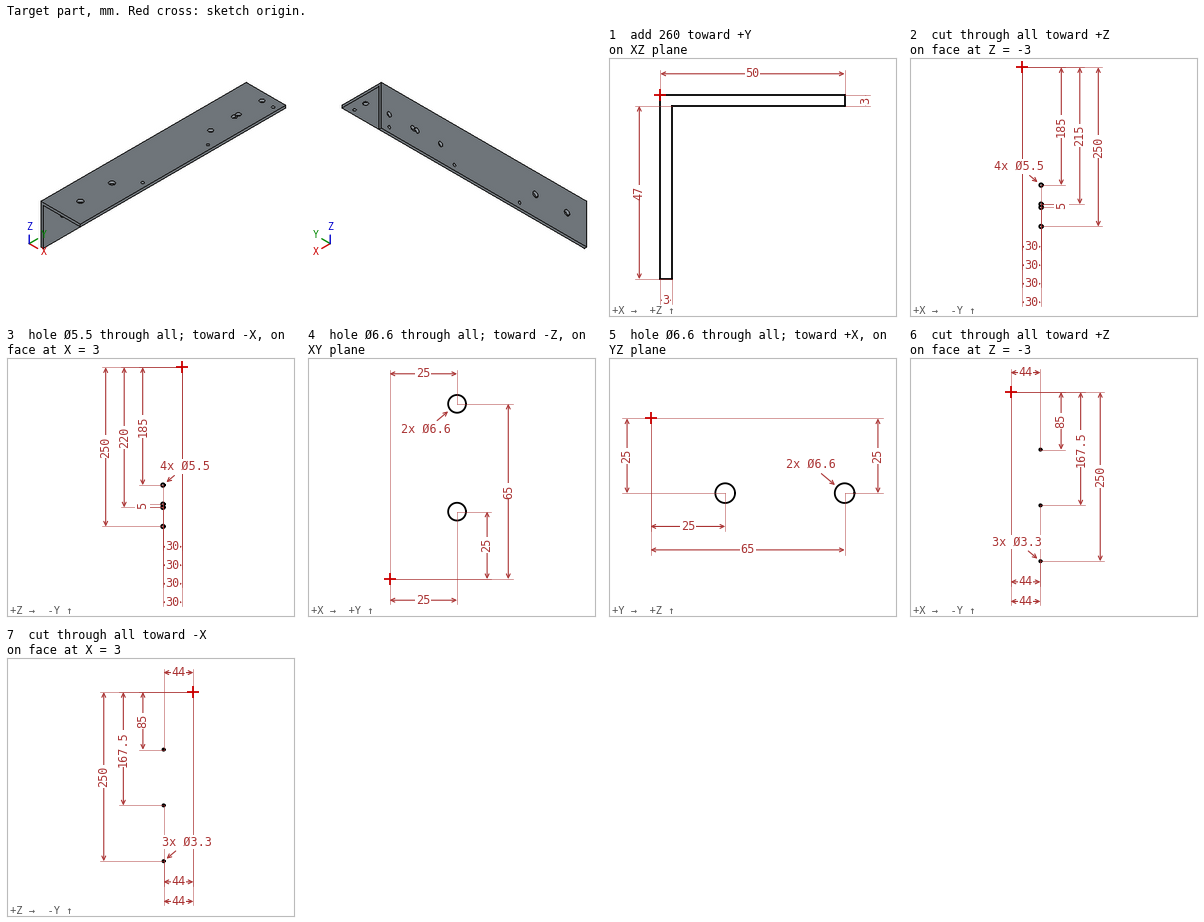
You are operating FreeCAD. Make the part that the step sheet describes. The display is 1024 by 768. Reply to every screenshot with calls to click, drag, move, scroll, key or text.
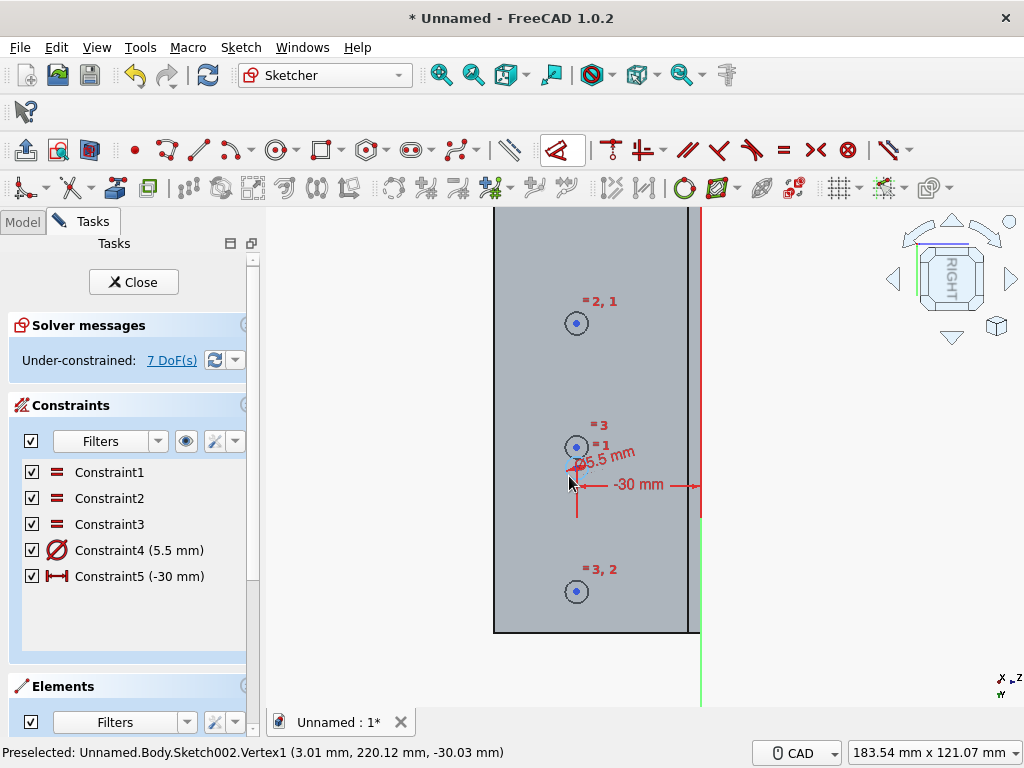
click(577, 324)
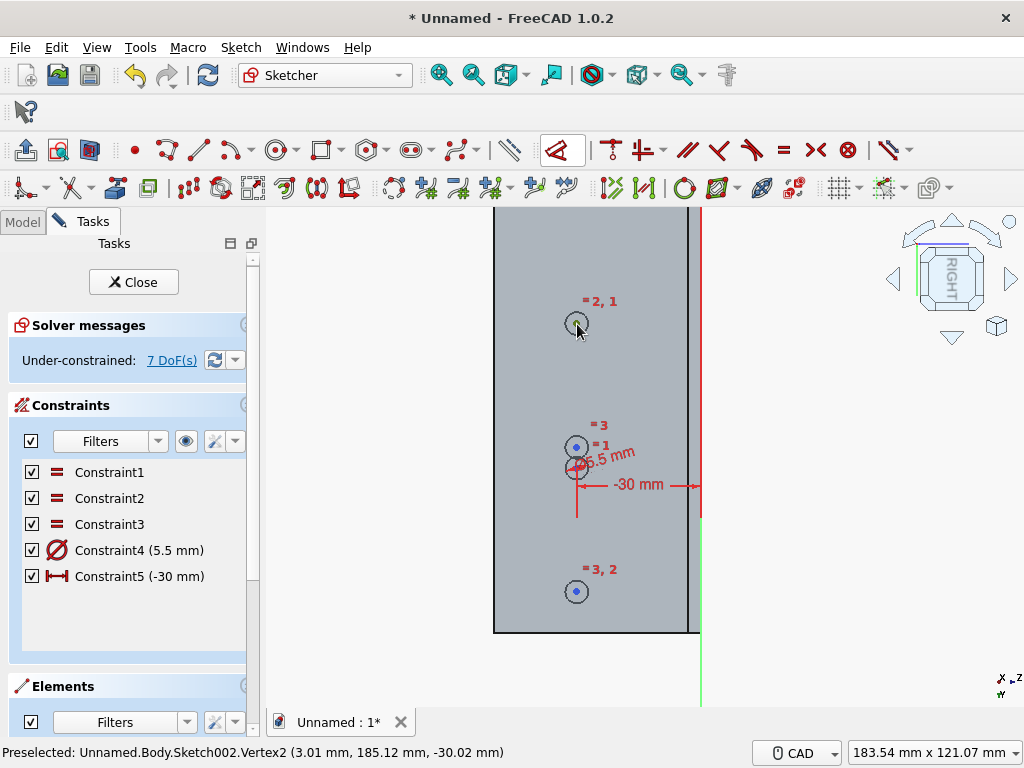
key(l)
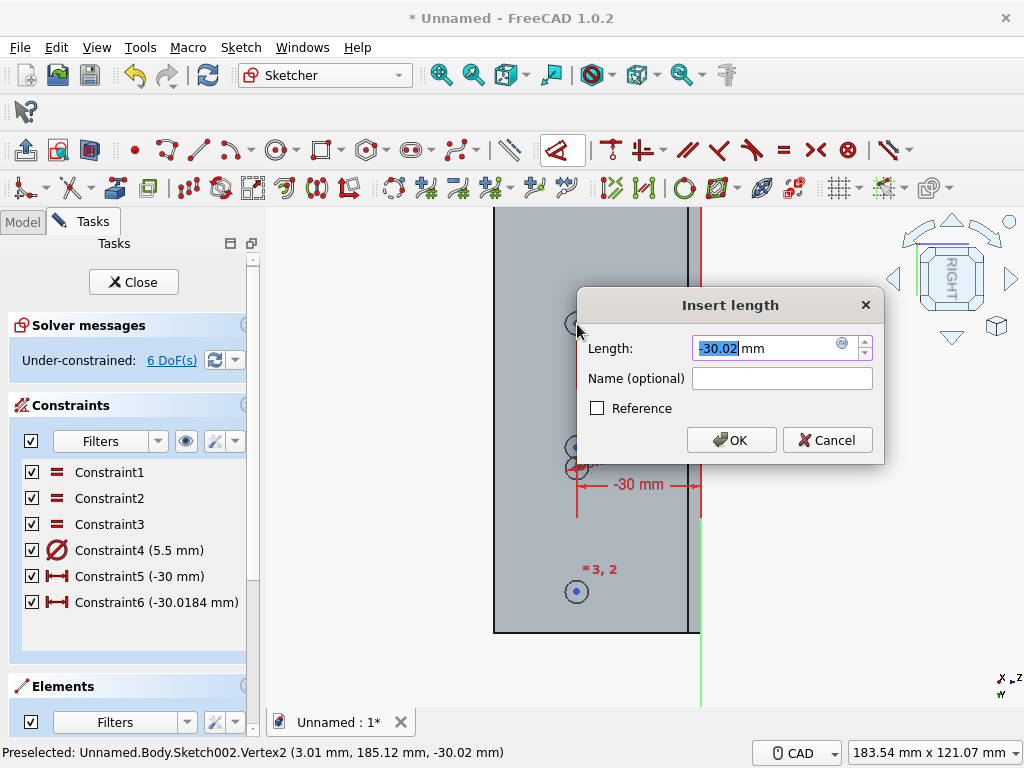
text(-30)
key(Return)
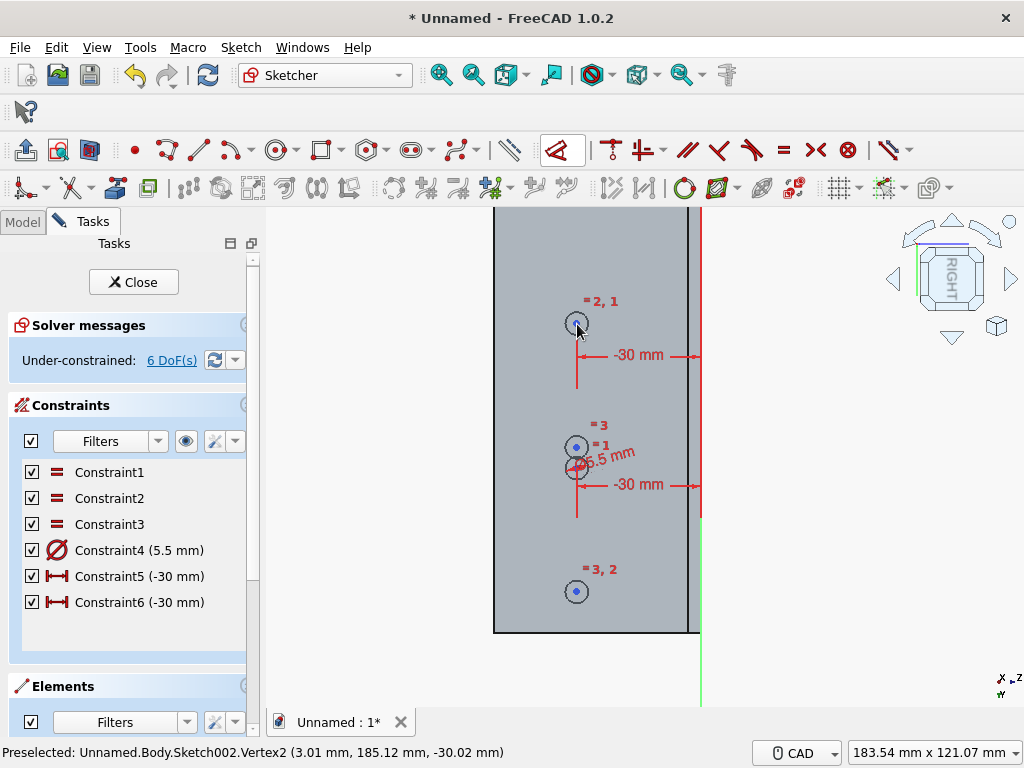
click(577, 592)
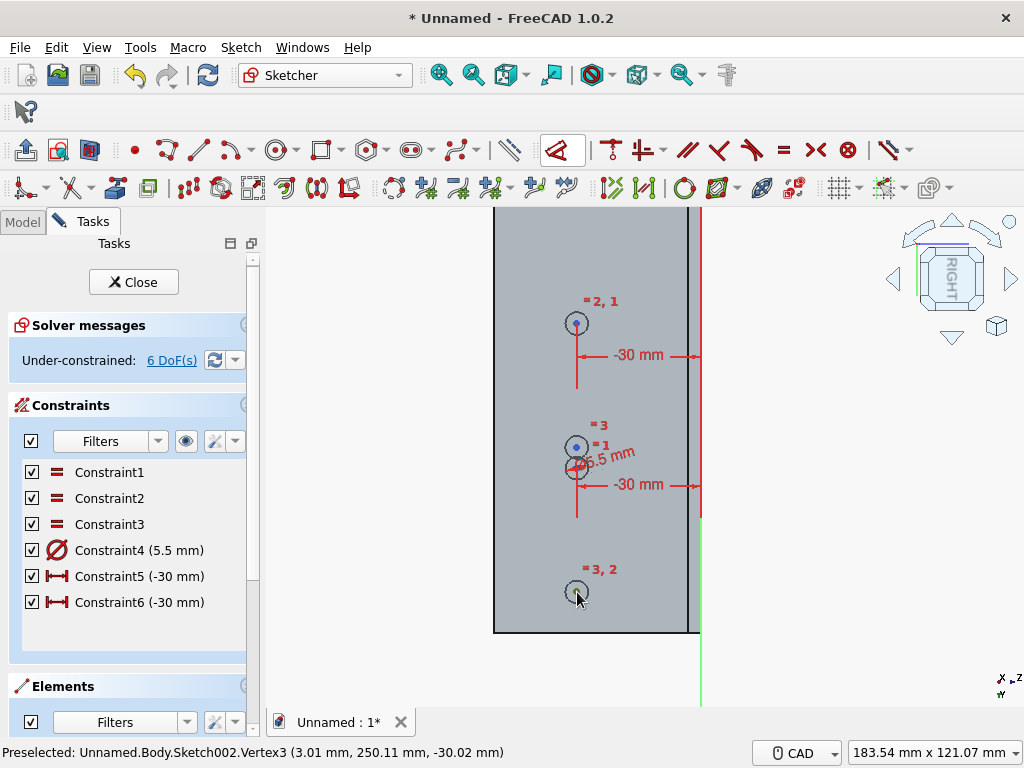
key(l)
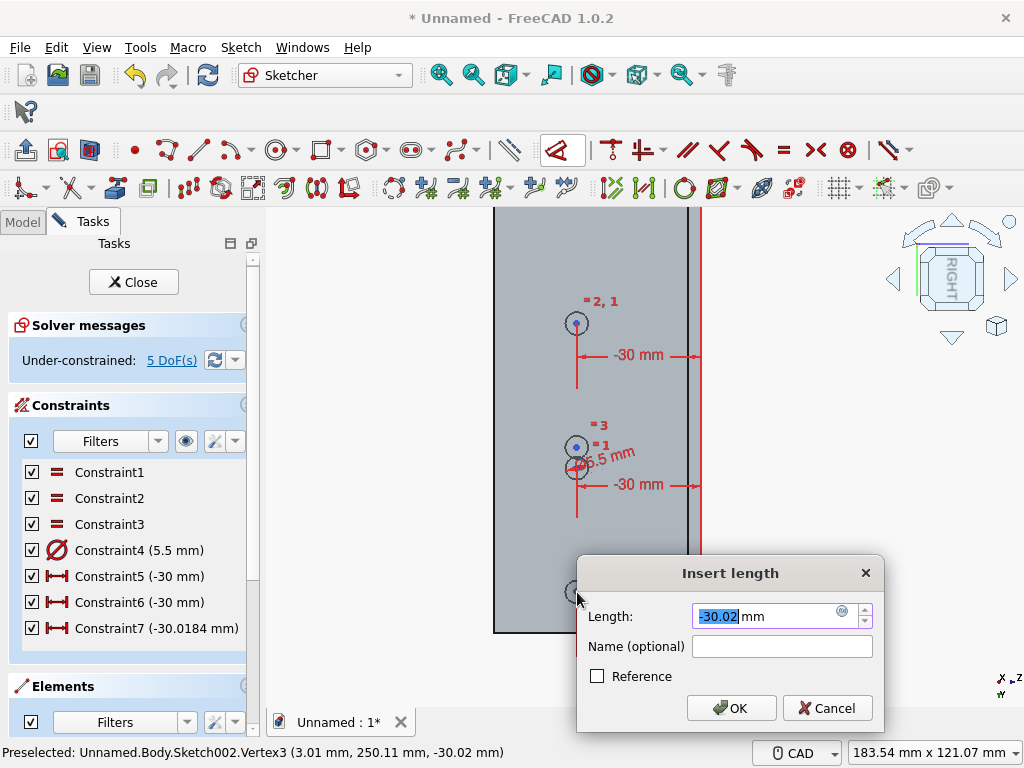
text(-30)
key(Return)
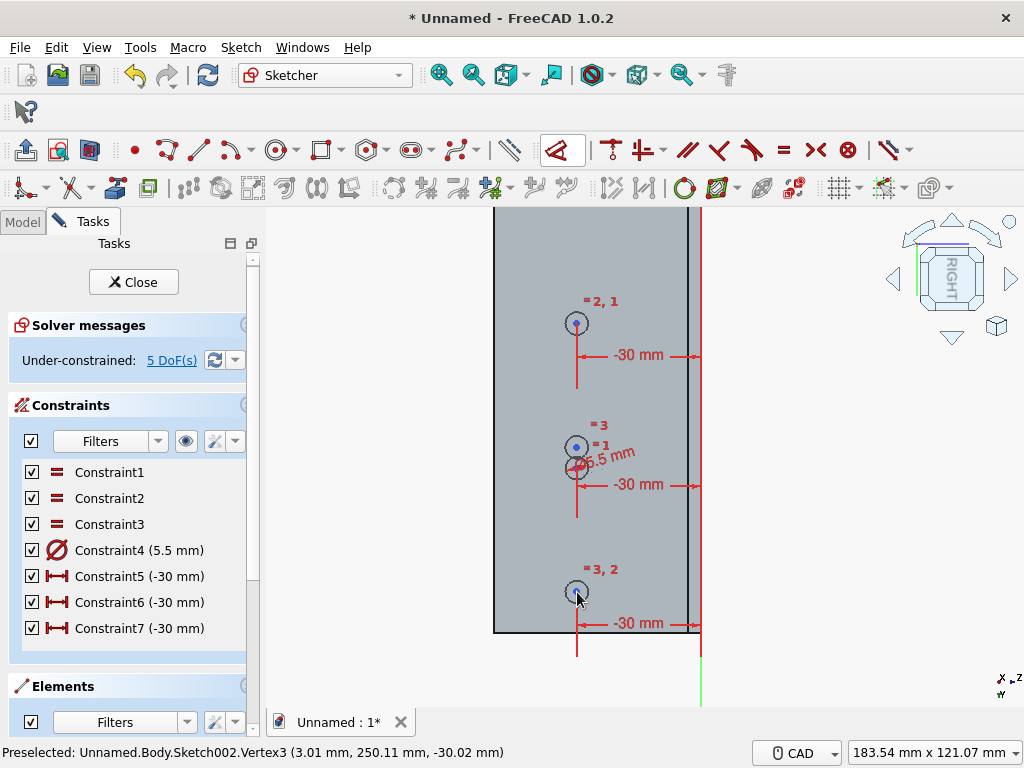
click(577, 447)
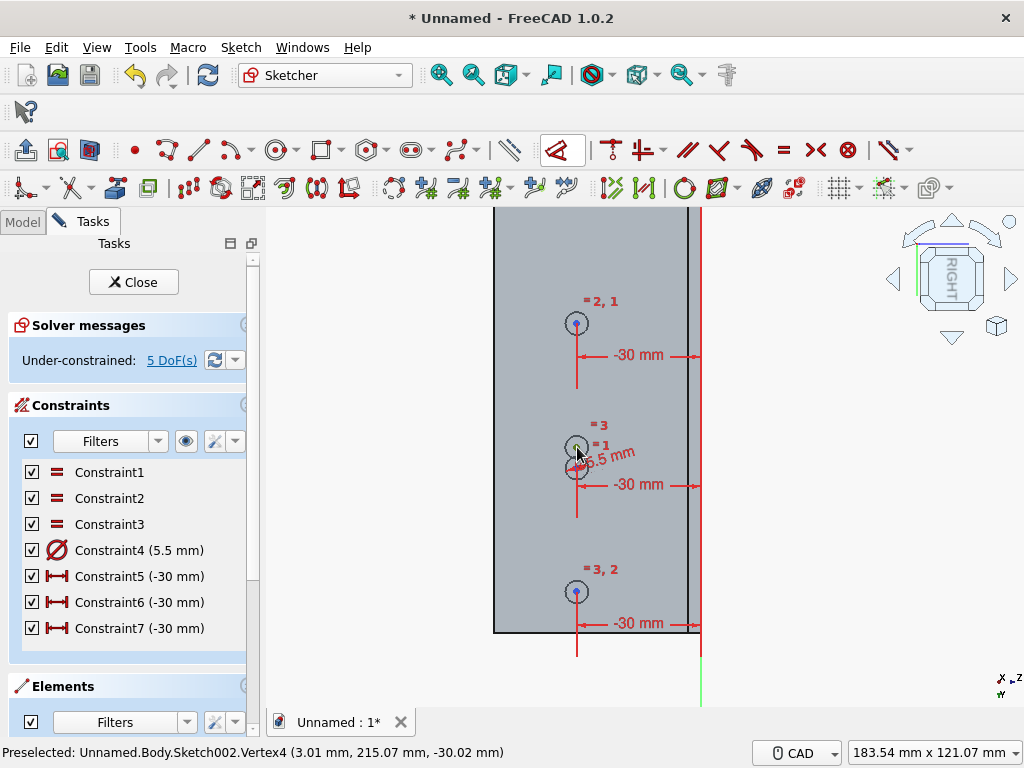
key(l)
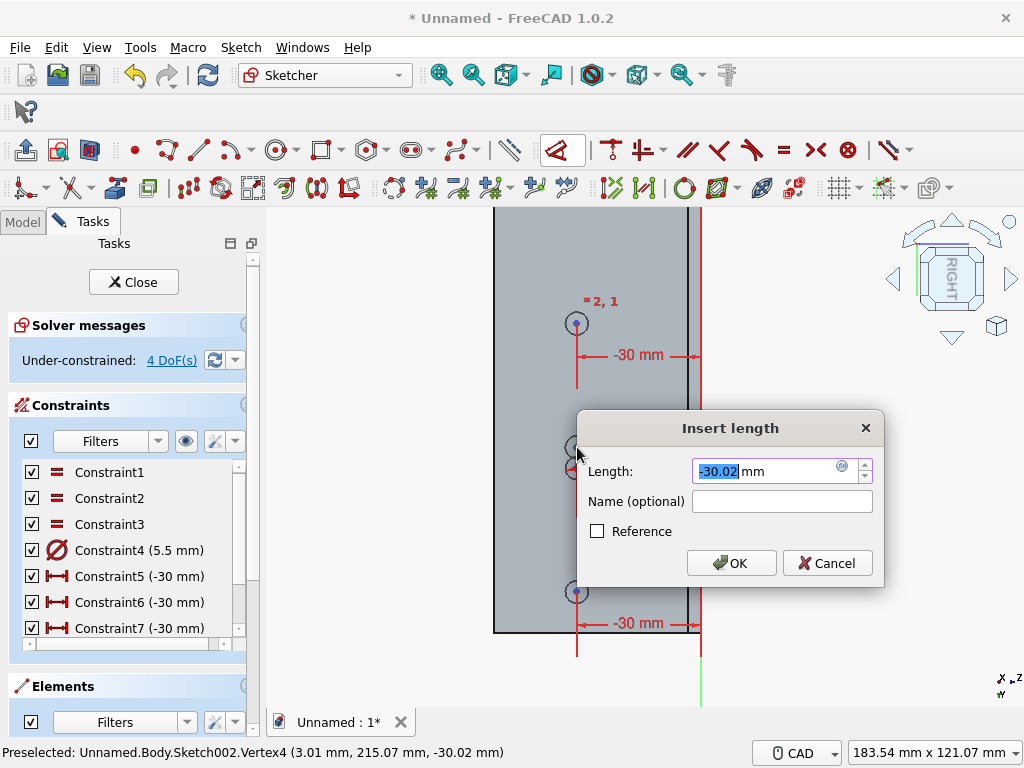
text(-30)
key(Return)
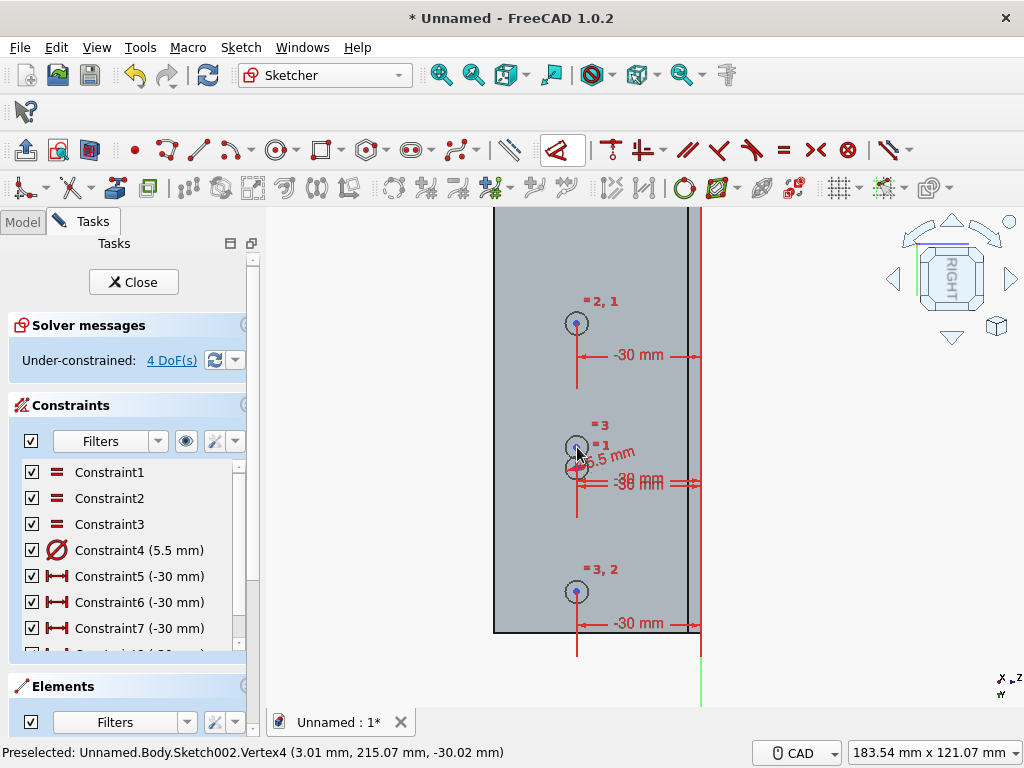
scroll(577, 468, up, 4)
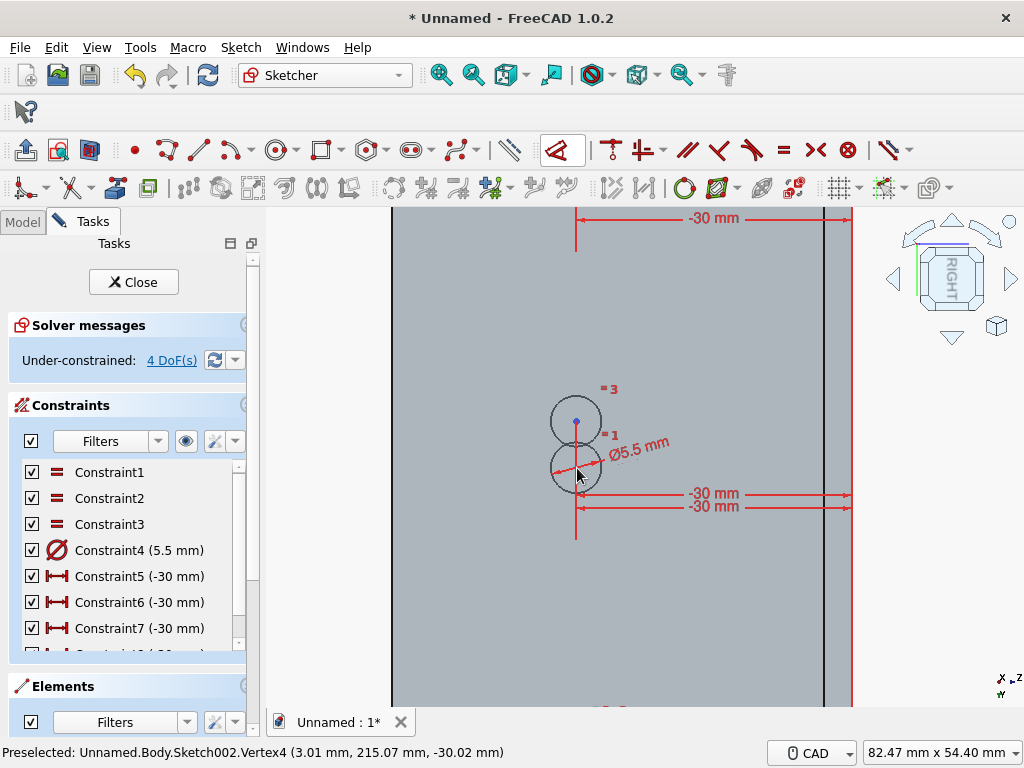
click(576, 468)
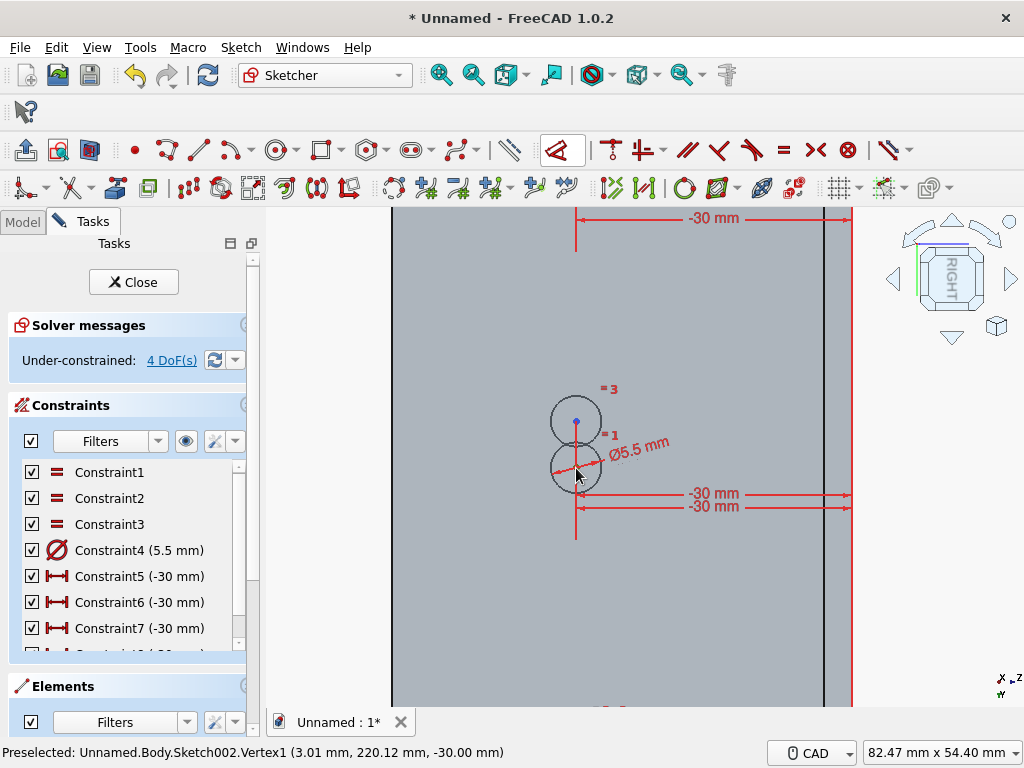
click(576, 421)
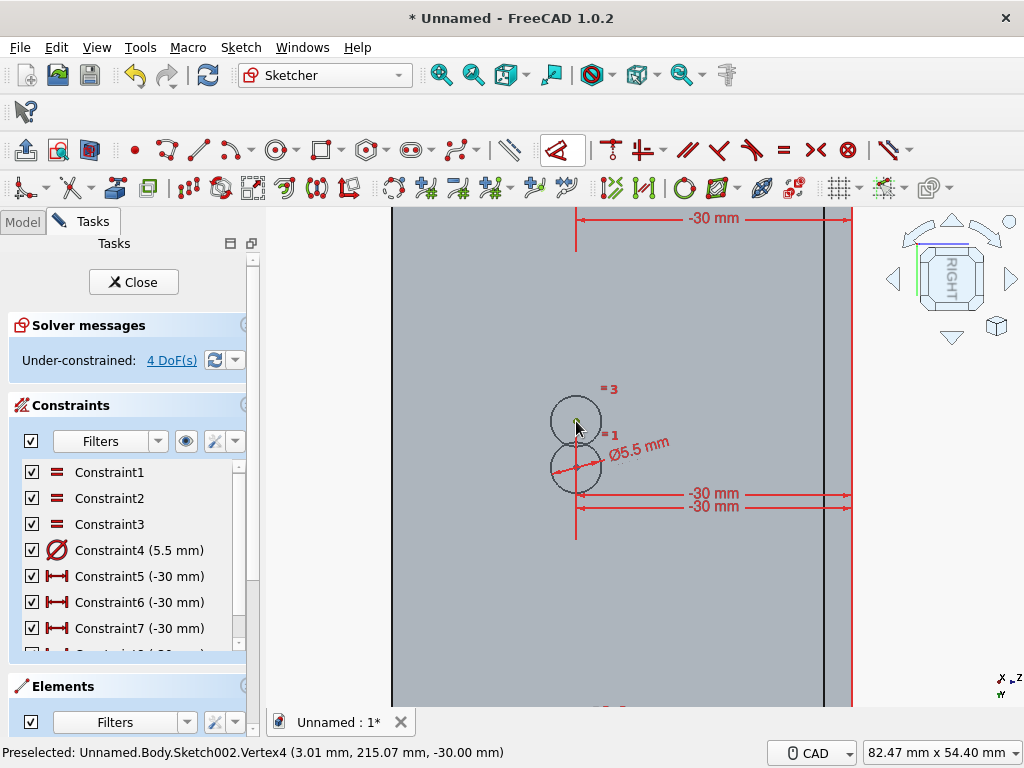
key(i)